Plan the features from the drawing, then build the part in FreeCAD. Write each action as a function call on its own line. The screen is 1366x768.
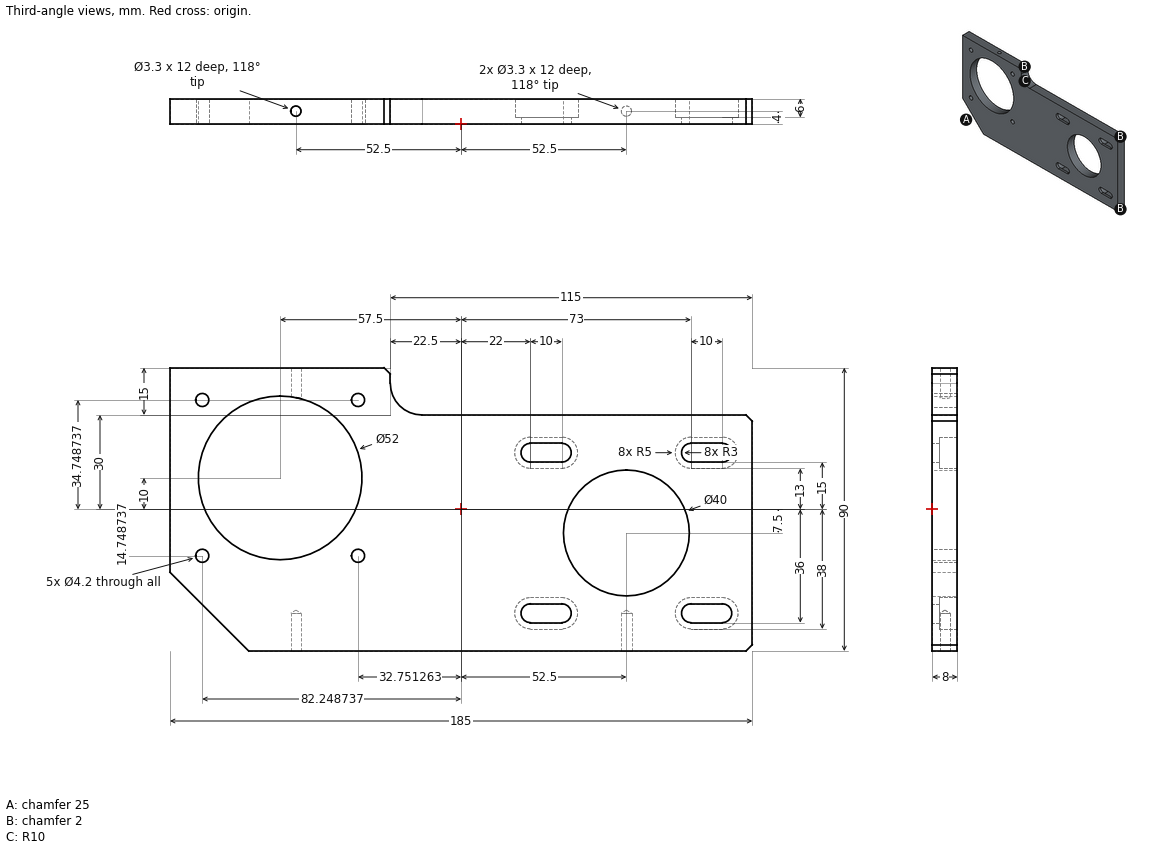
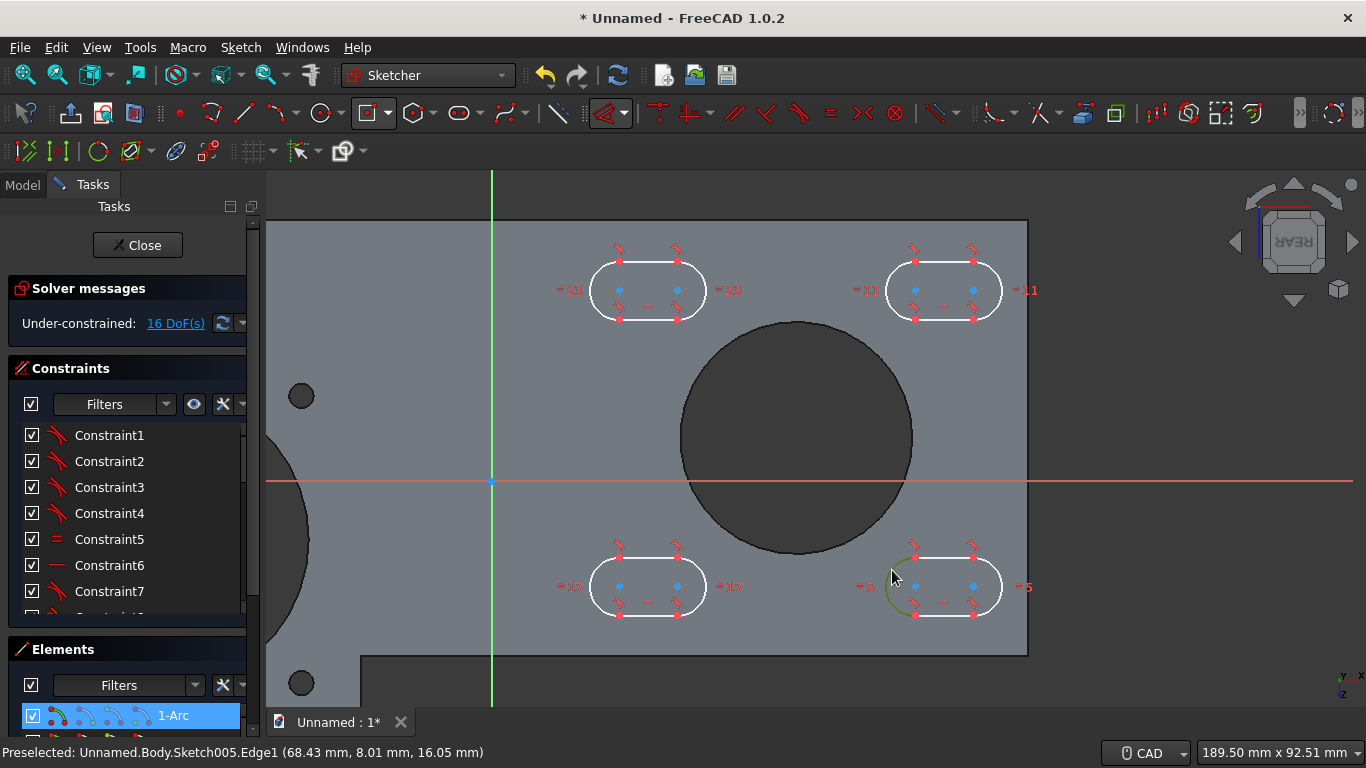
click(892, 274)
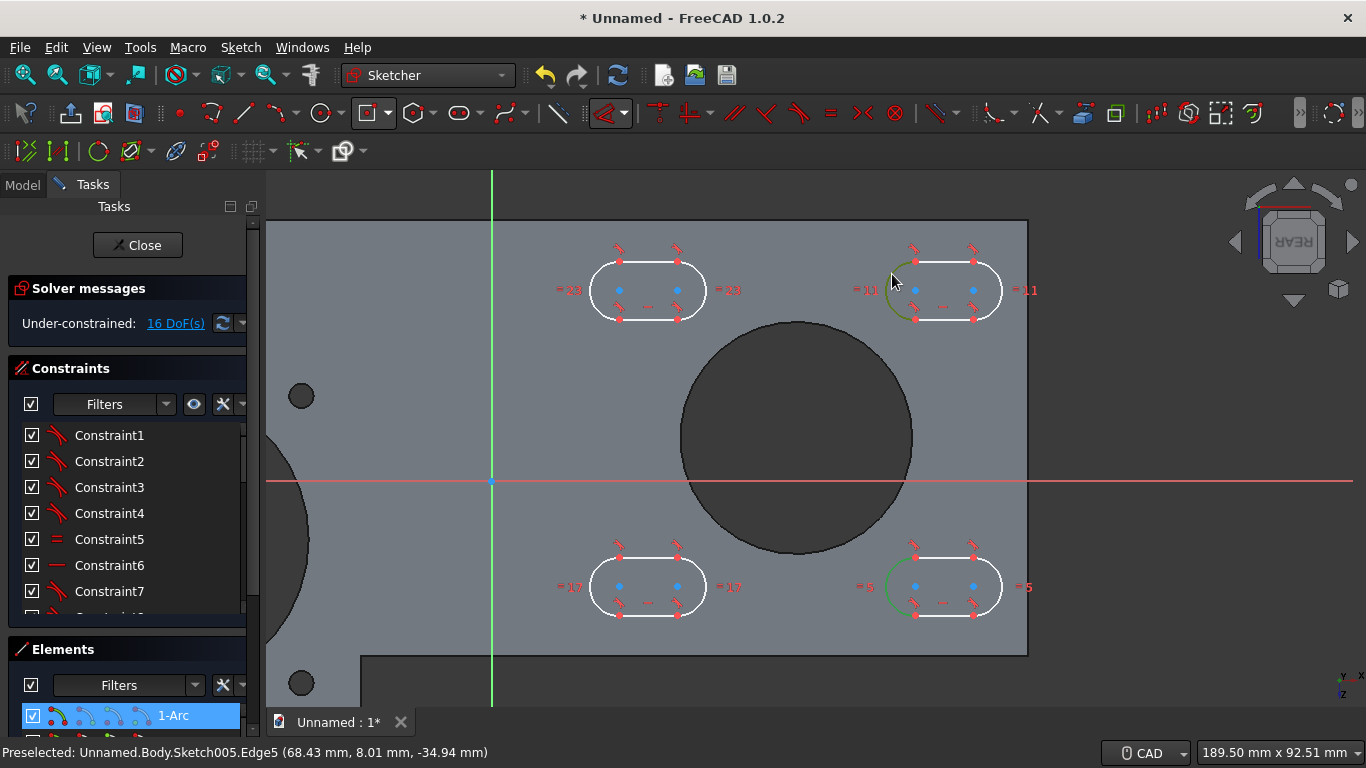
click(596, 570)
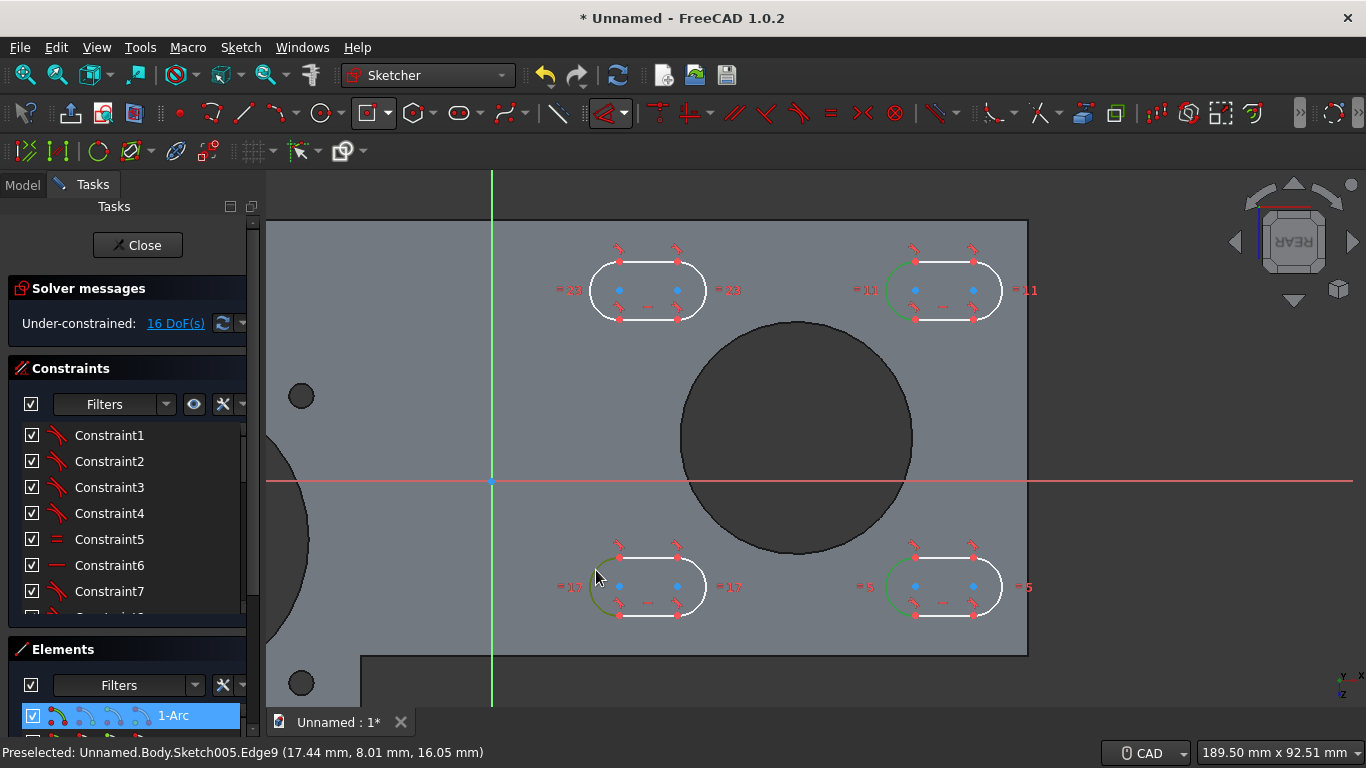
click(596, 274)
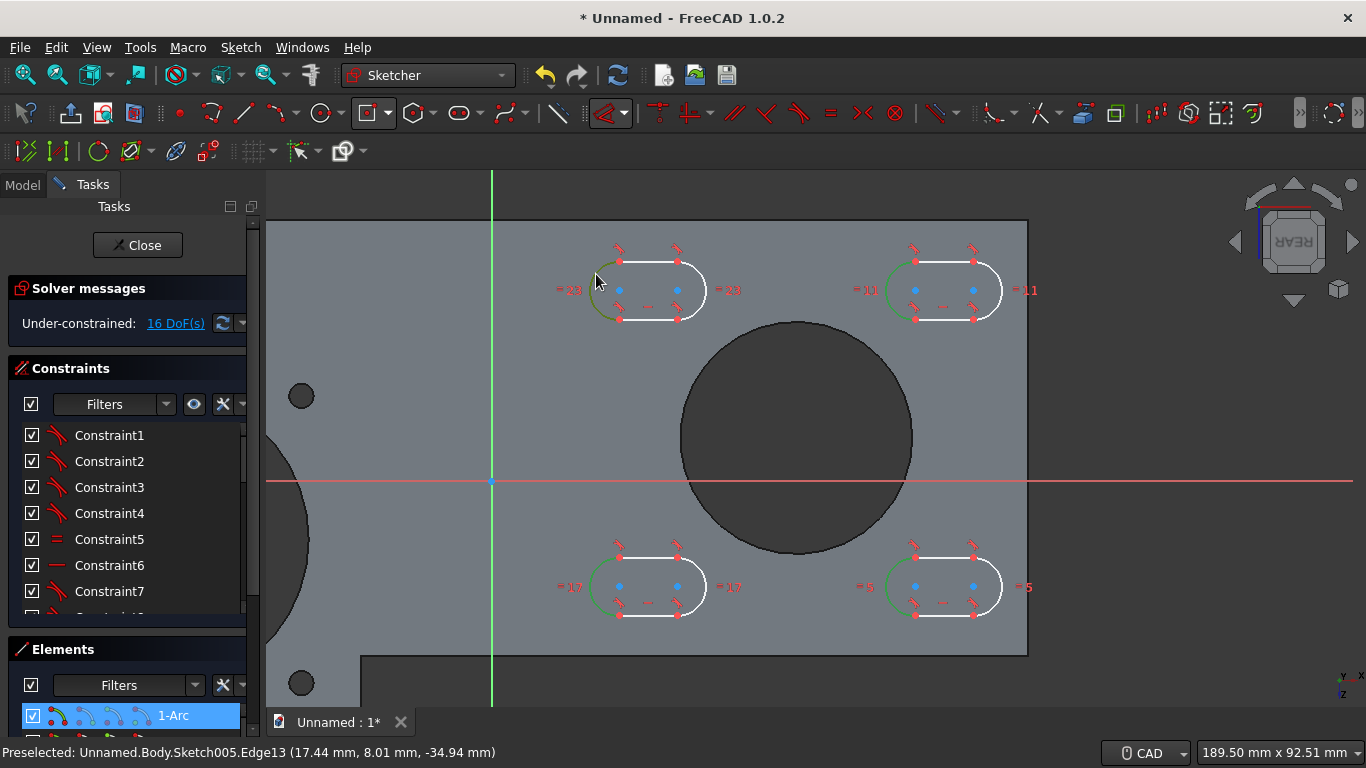
click(832, 114)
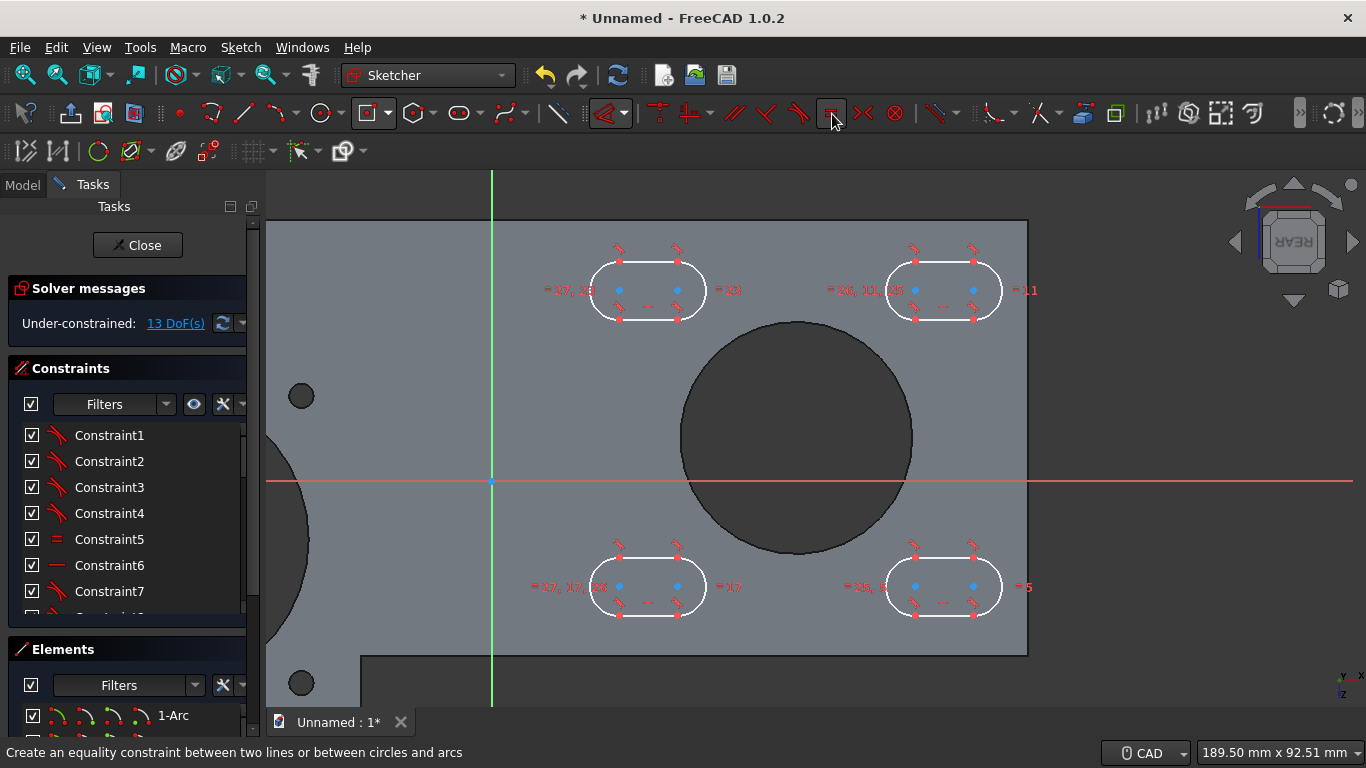
scroll(892, 570, up, 2)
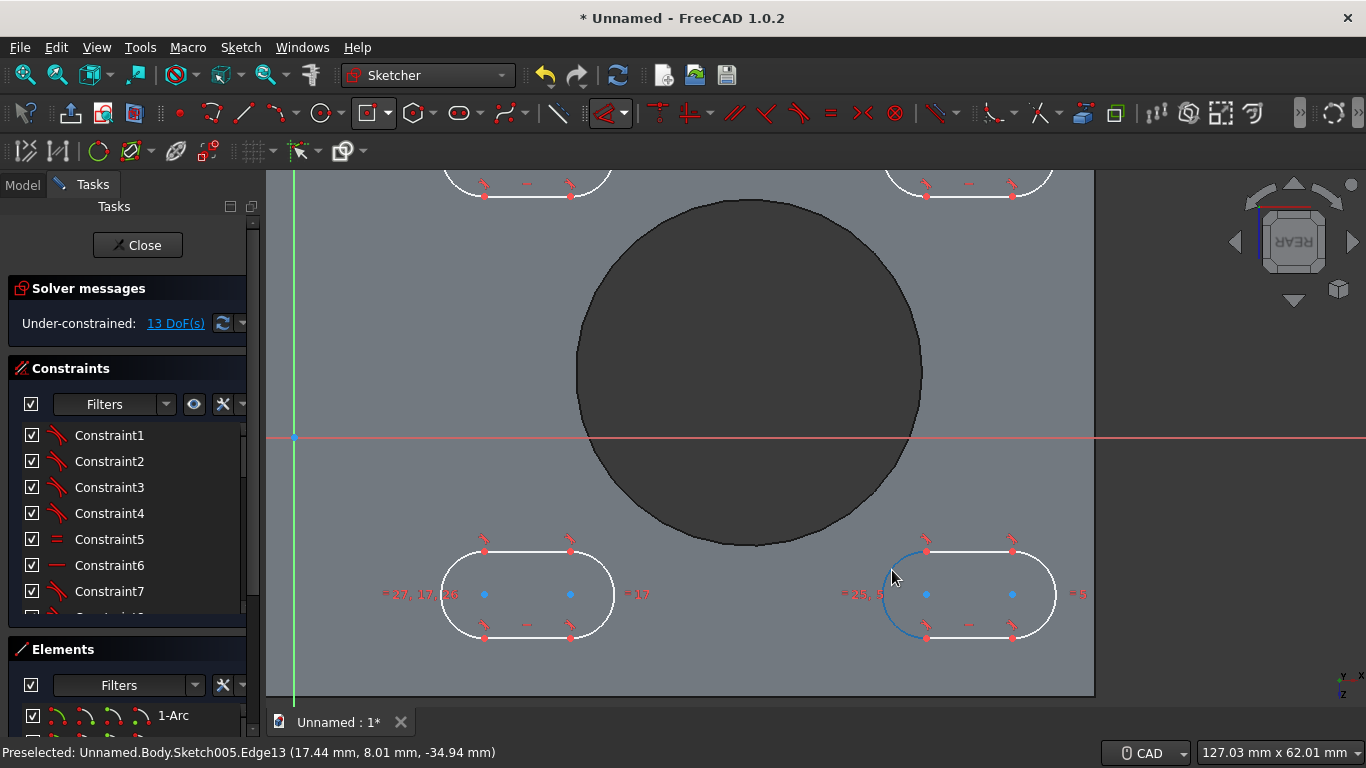
click(891, 570)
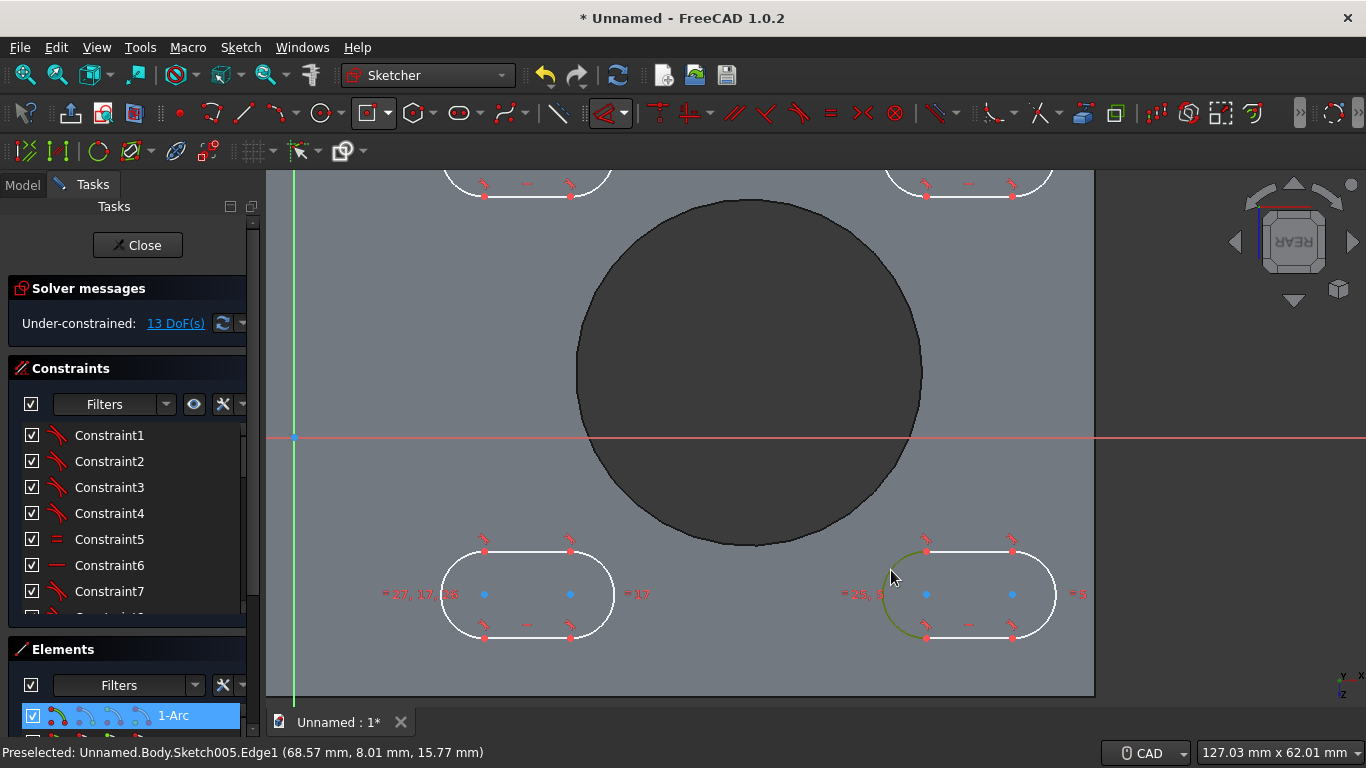
click(626, 114)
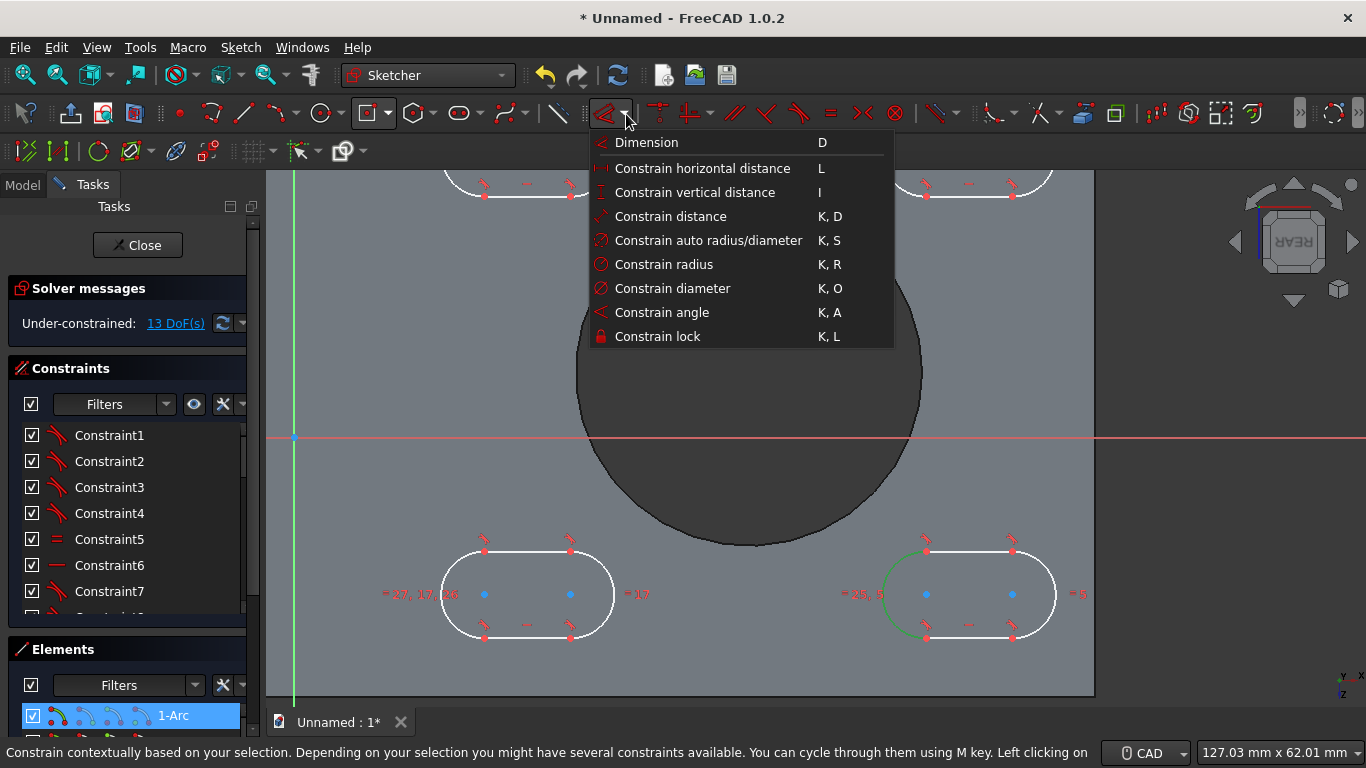
click(742, 264)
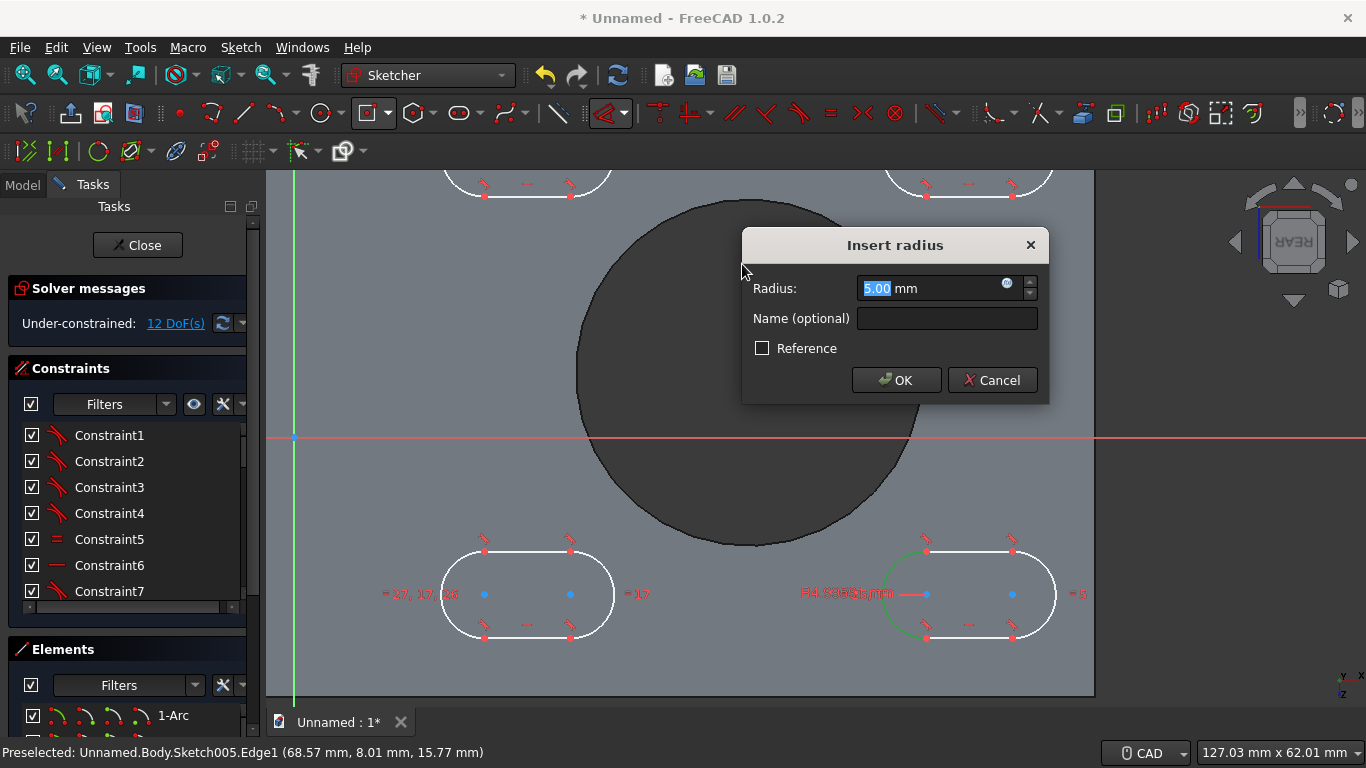
text(5)
key(Return)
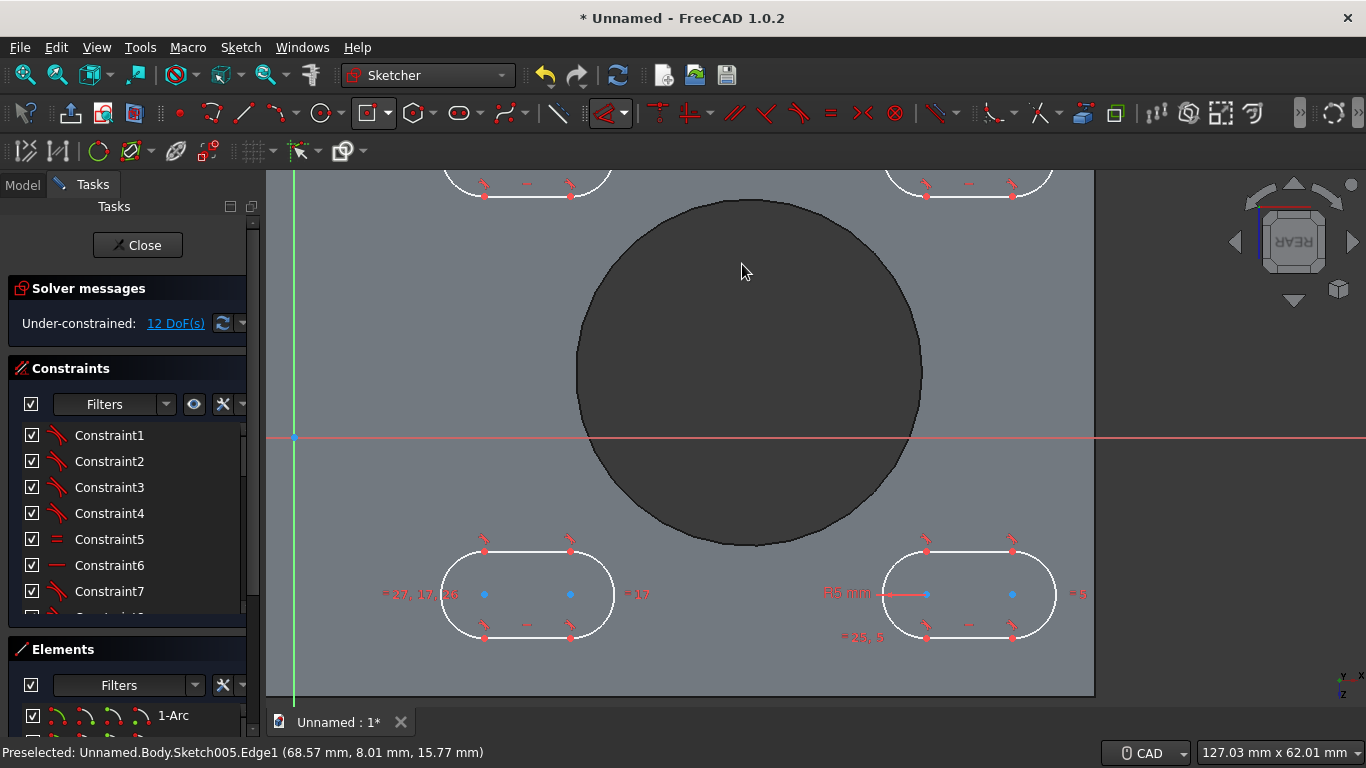
click(952, 552)